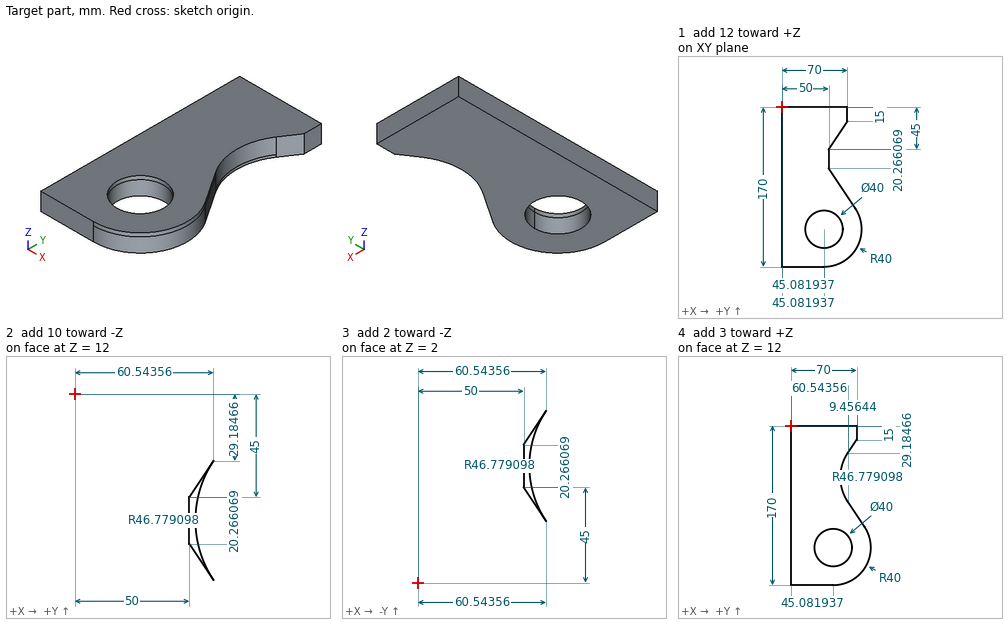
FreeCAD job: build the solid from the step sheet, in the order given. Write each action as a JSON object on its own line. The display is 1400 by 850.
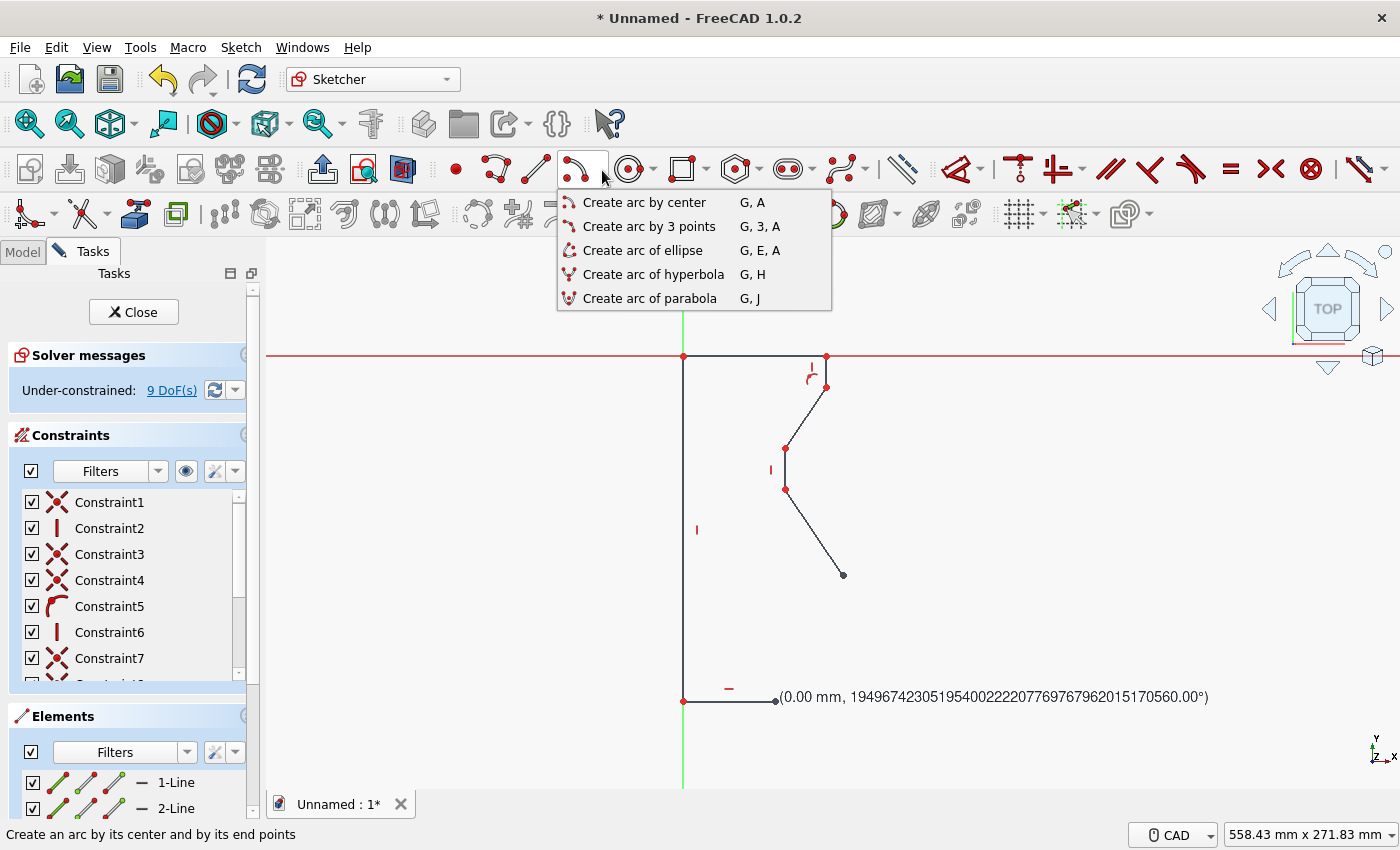
{"action": "left_click", "coordinate": [694, 226]}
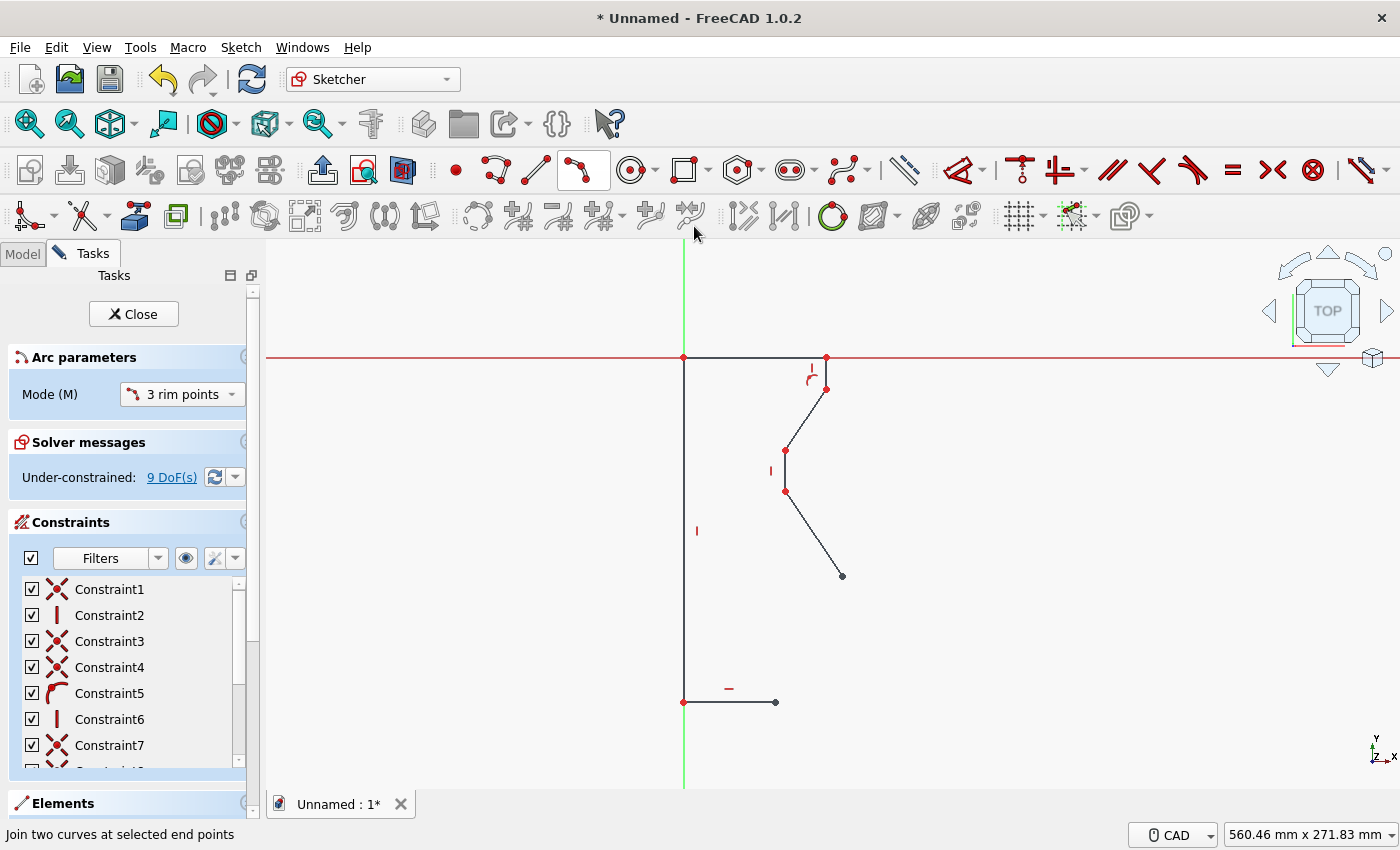
{"action": "left_click", "coordinate": [775, 702]}
{"action": "left_click", "coordinate": [843, 577]}
{"action": "left_click", "coordinate": [846, 659]}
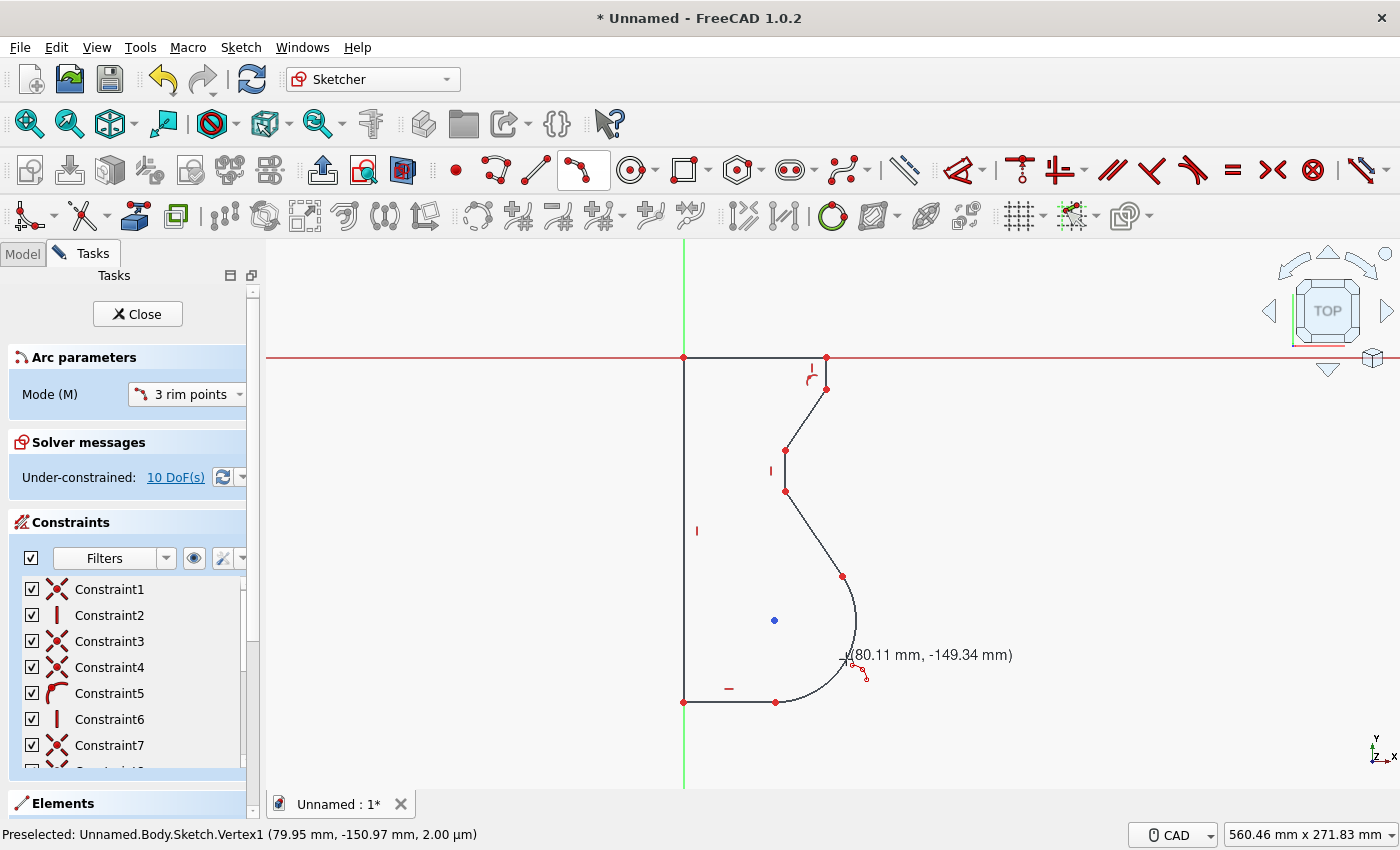
{"action": "left_click", "coordinate": [632, 170]}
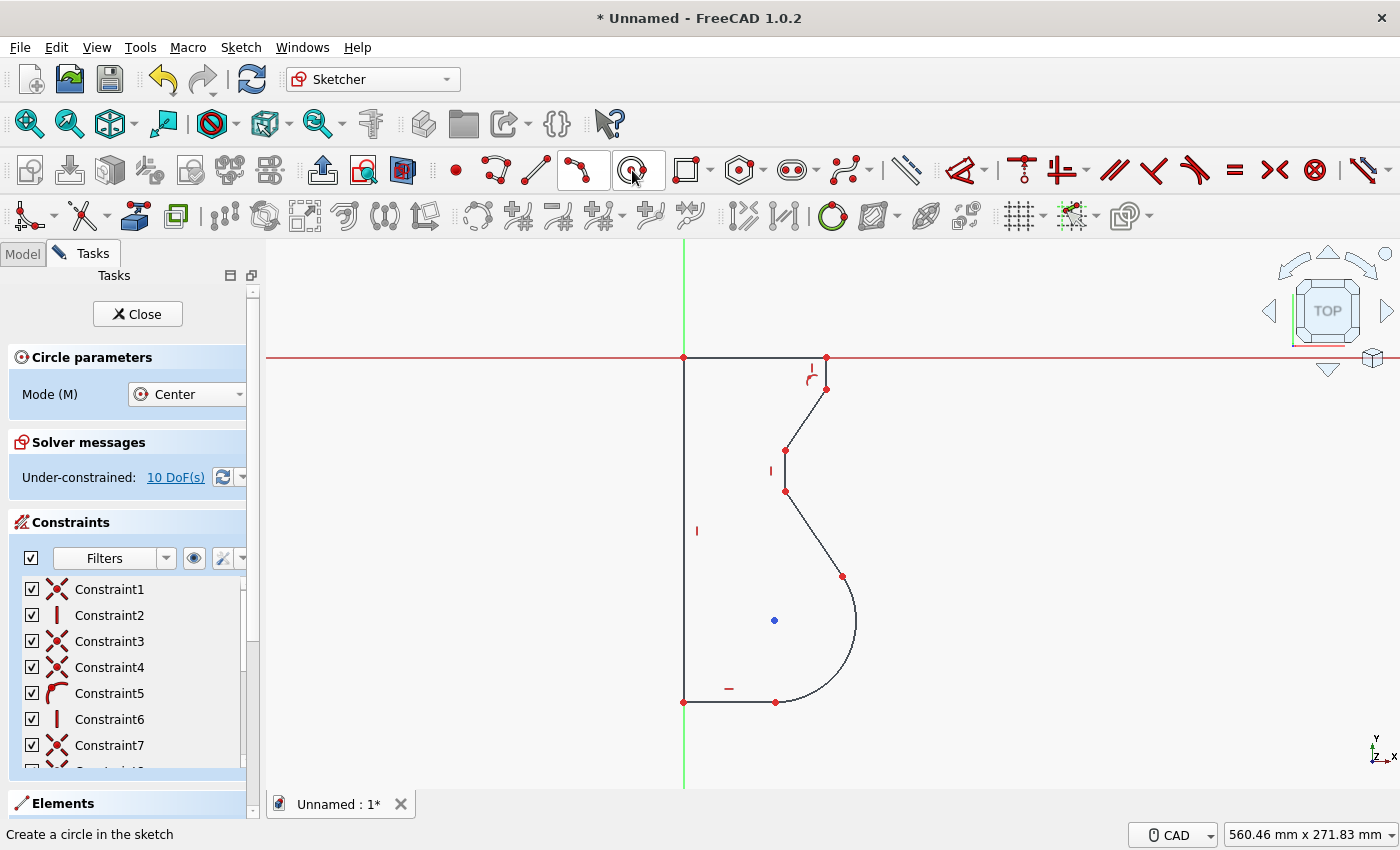
{"action": "left_click", "coordinate": [775, 621]}
{"action": "left_click", "coordinate": [804, 592]}
{"action": "key", "text": "Escape"}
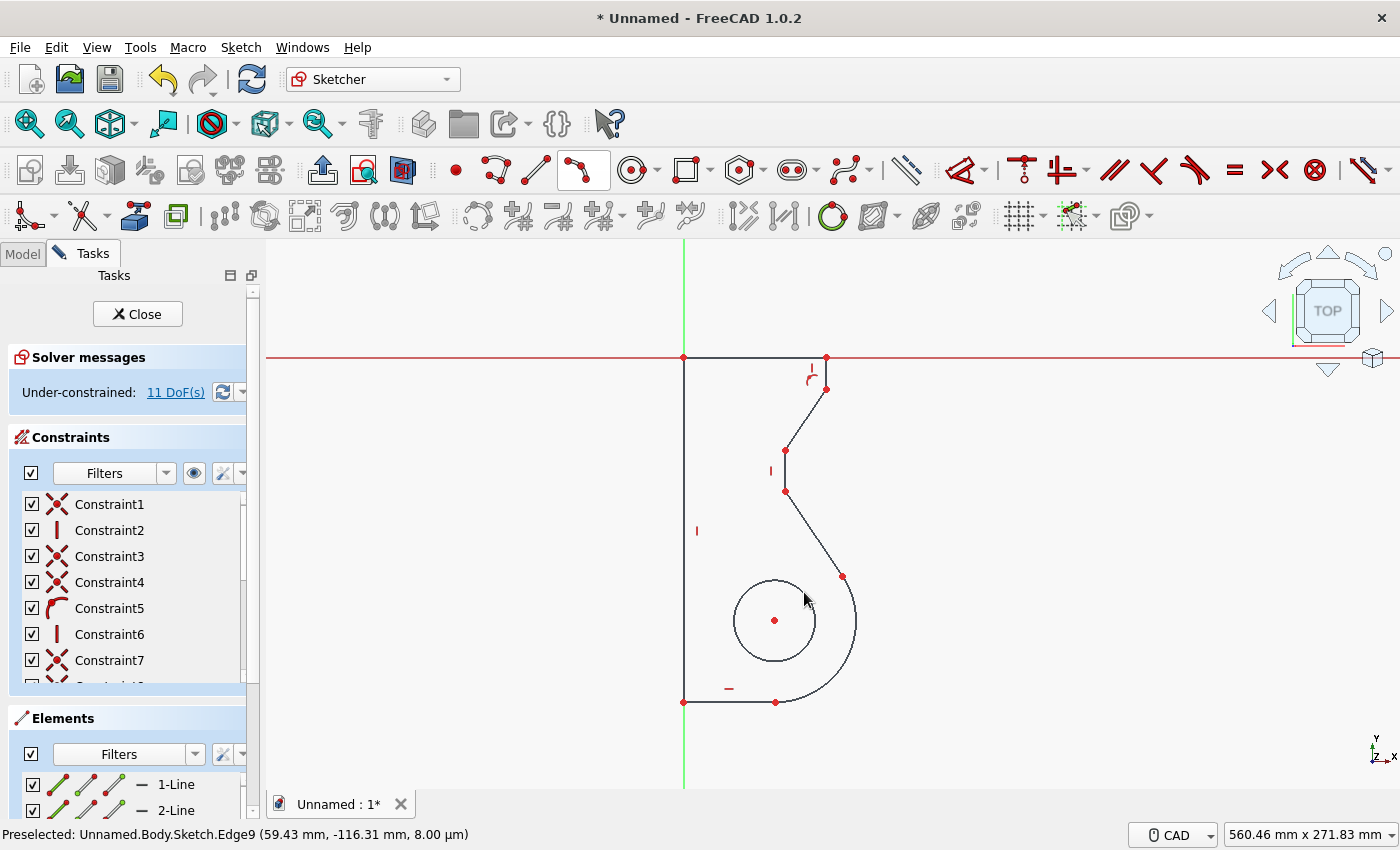
{"action": "left_click", "coordinate": [826, 551]}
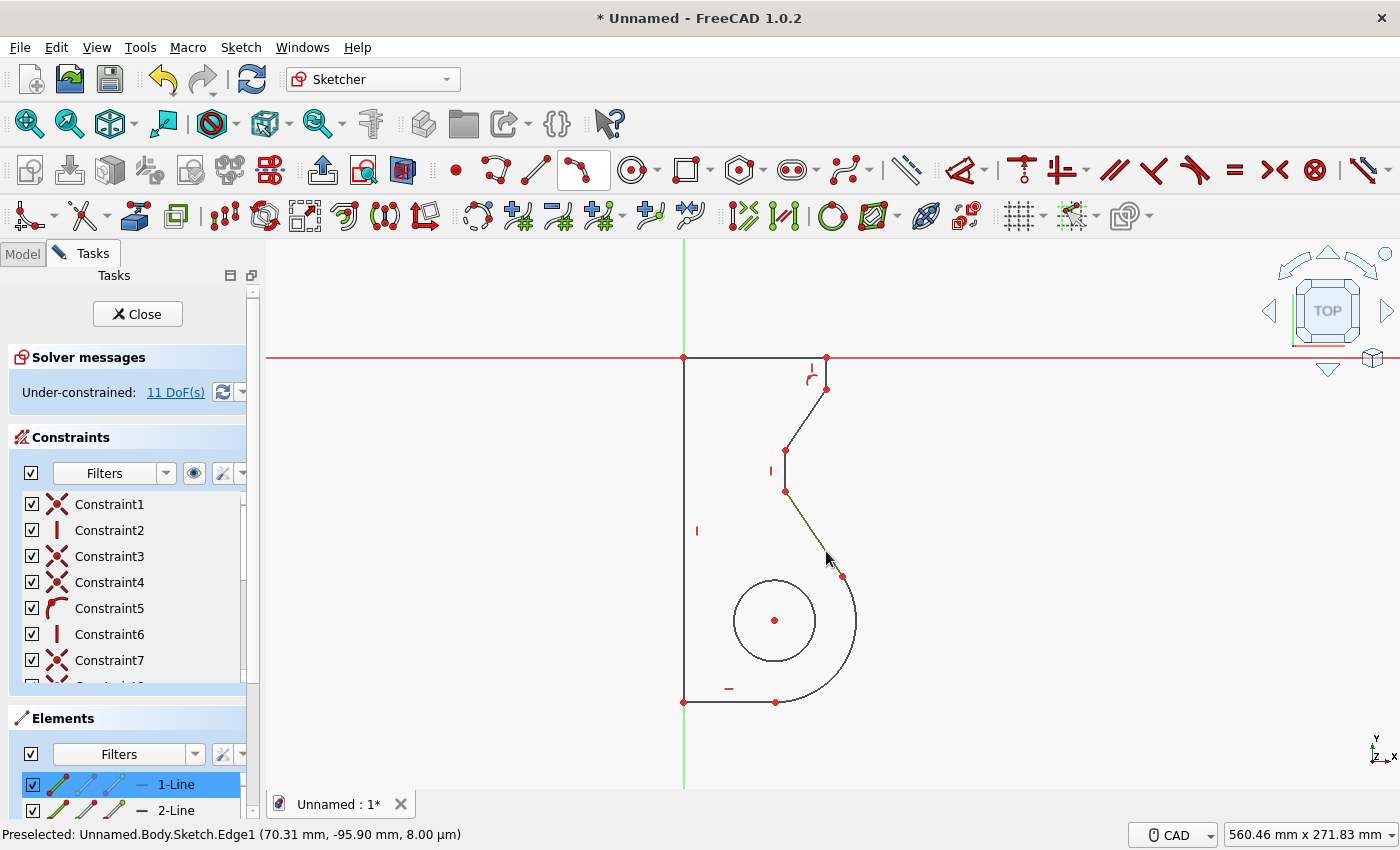
{"action": "left_click", "coordinate": [824, 686]}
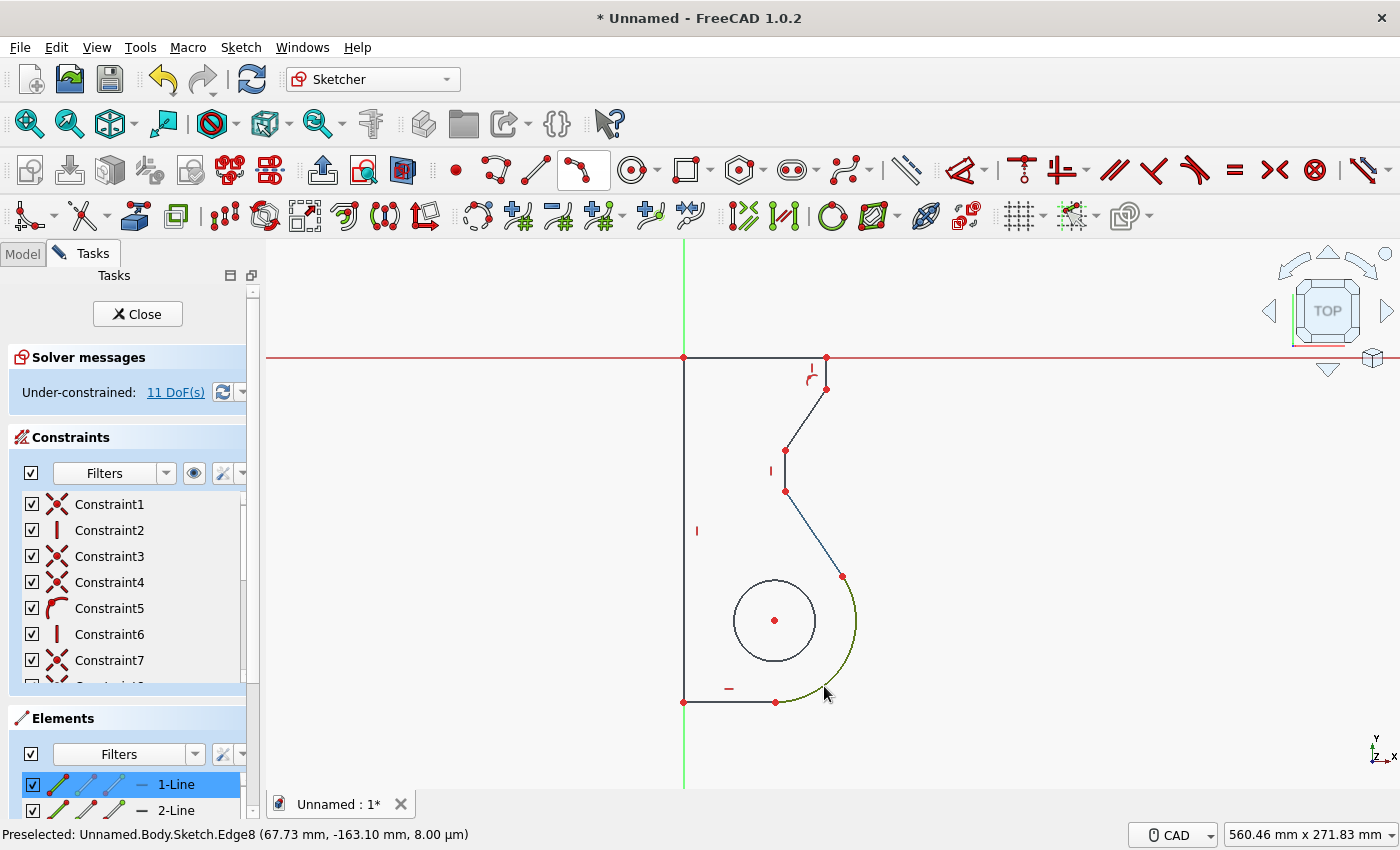
{"action": "left_click", "coordinate": [1196, 170]}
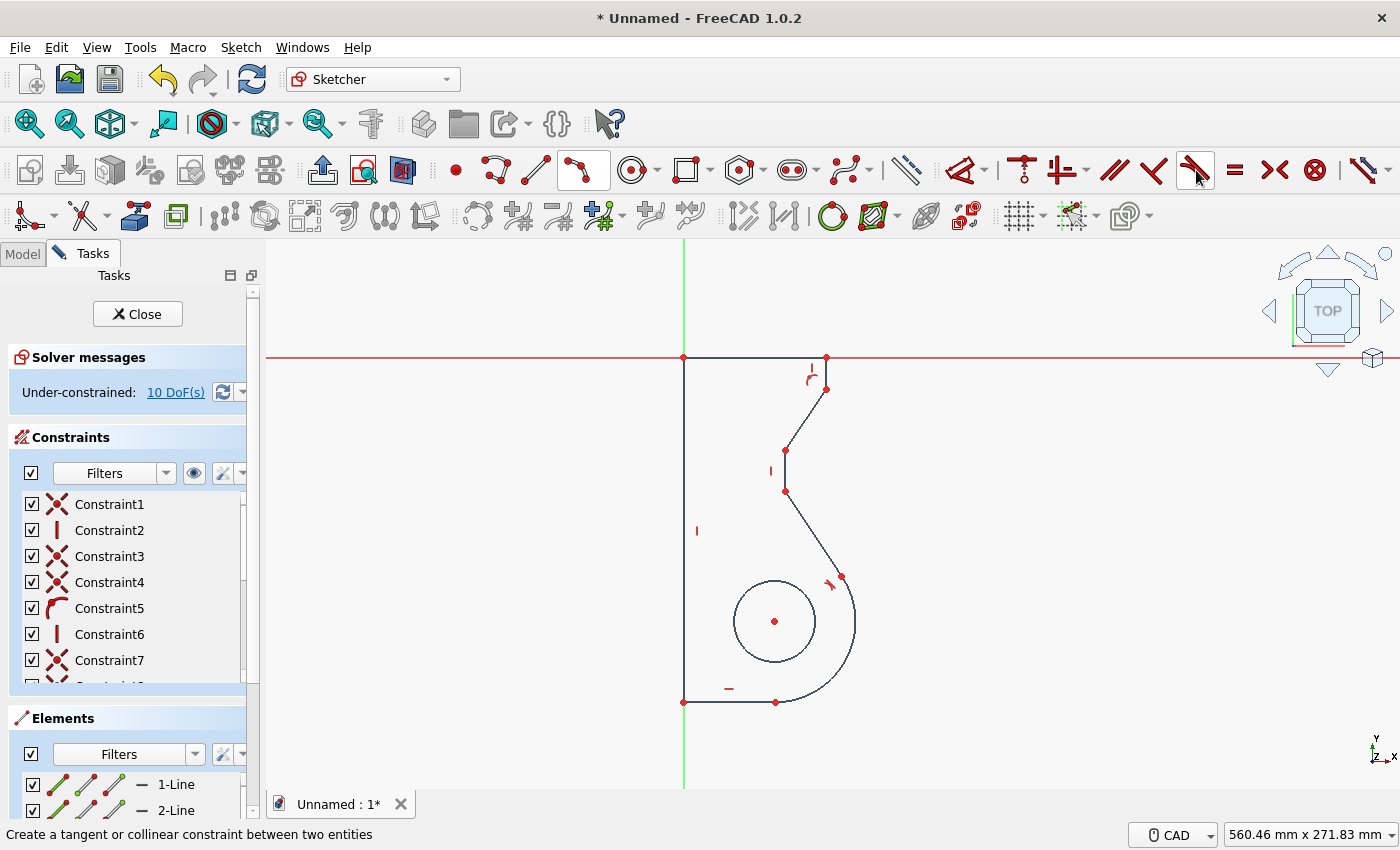
{"action": "left_click", "coordinate": [960, 170]}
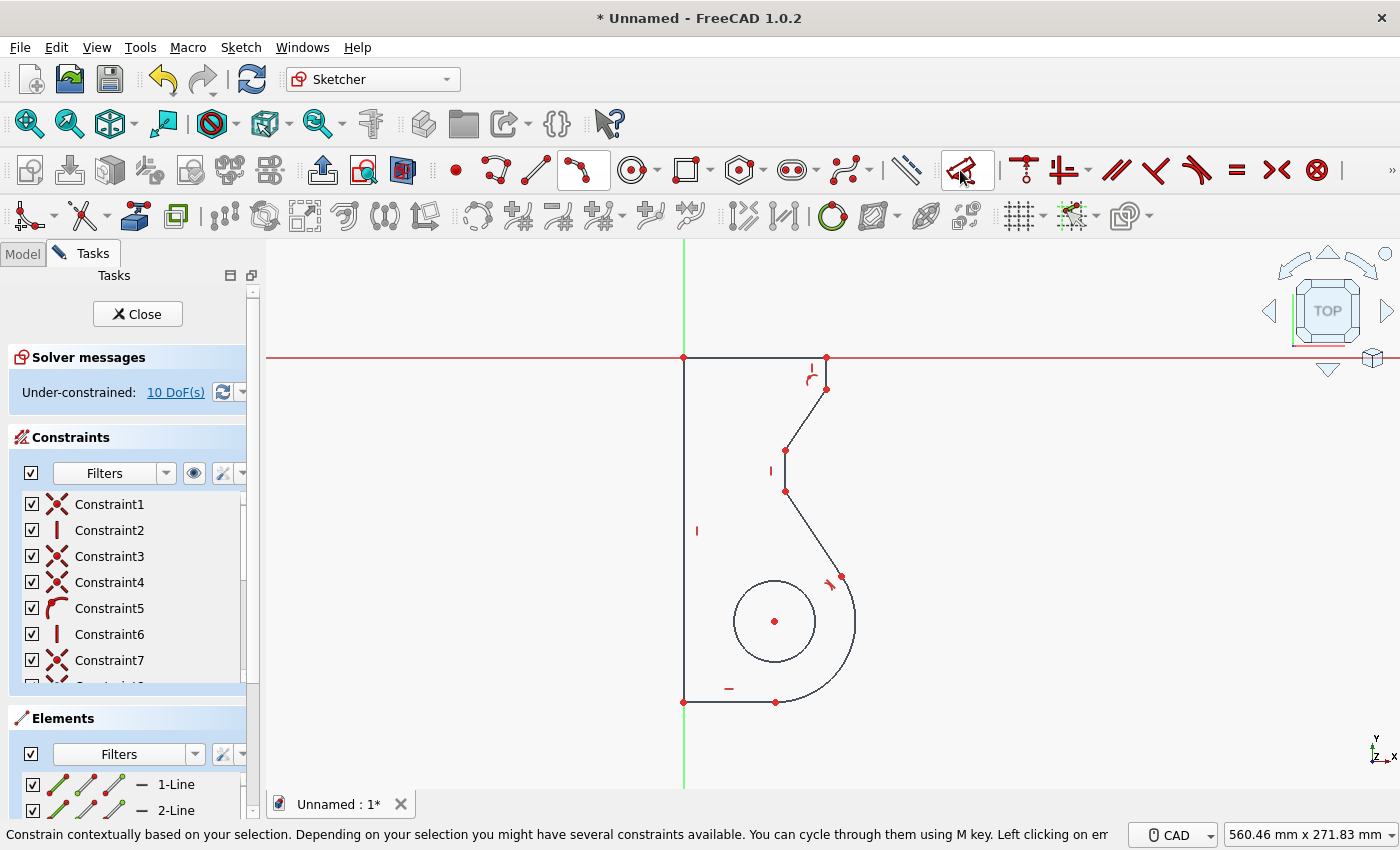
{"action": "left_click", "coordinate": [824, 686]}
{"action": "left_click", "coordinate": [843, 711]}